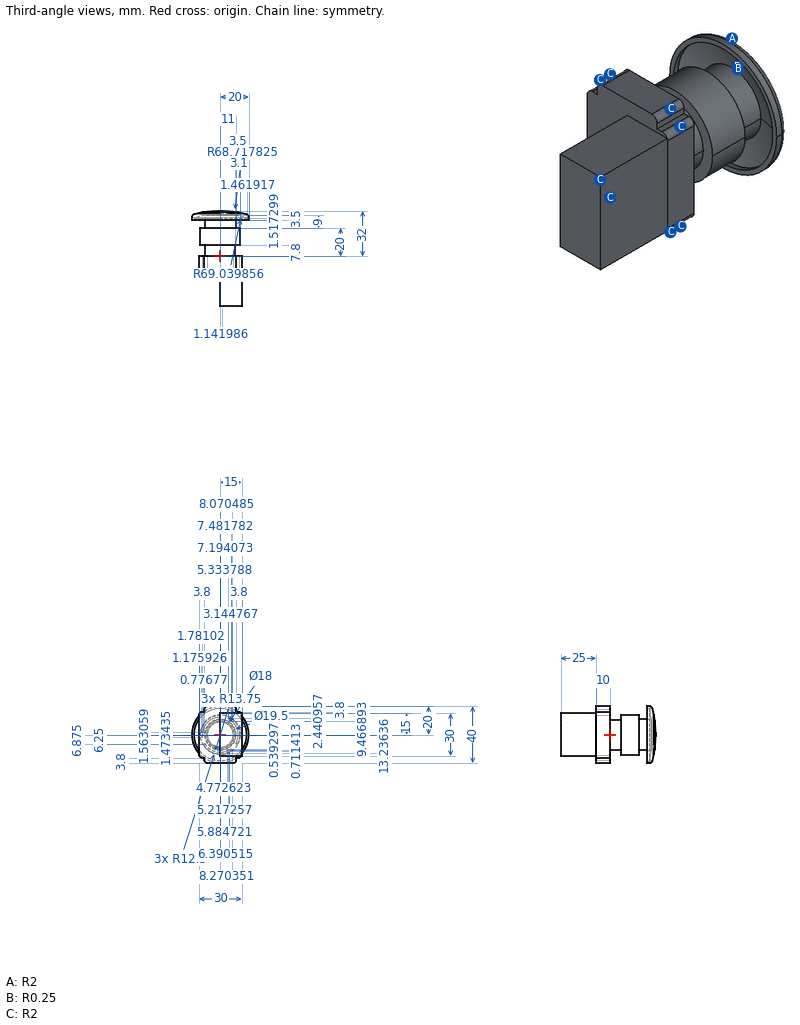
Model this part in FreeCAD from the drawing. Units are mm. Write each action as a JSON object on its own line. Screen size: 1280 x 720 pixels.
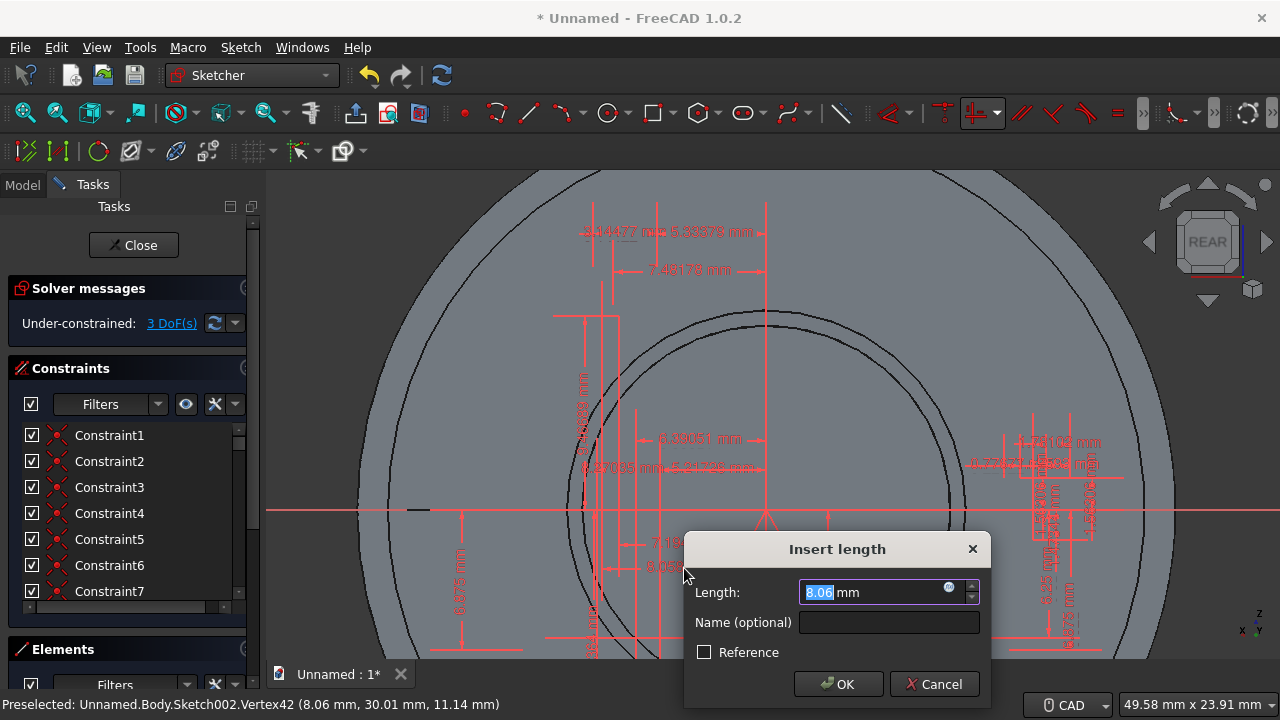
{"action": "type", "text": "8.070485"}
{"action": "key", "text": "Return"}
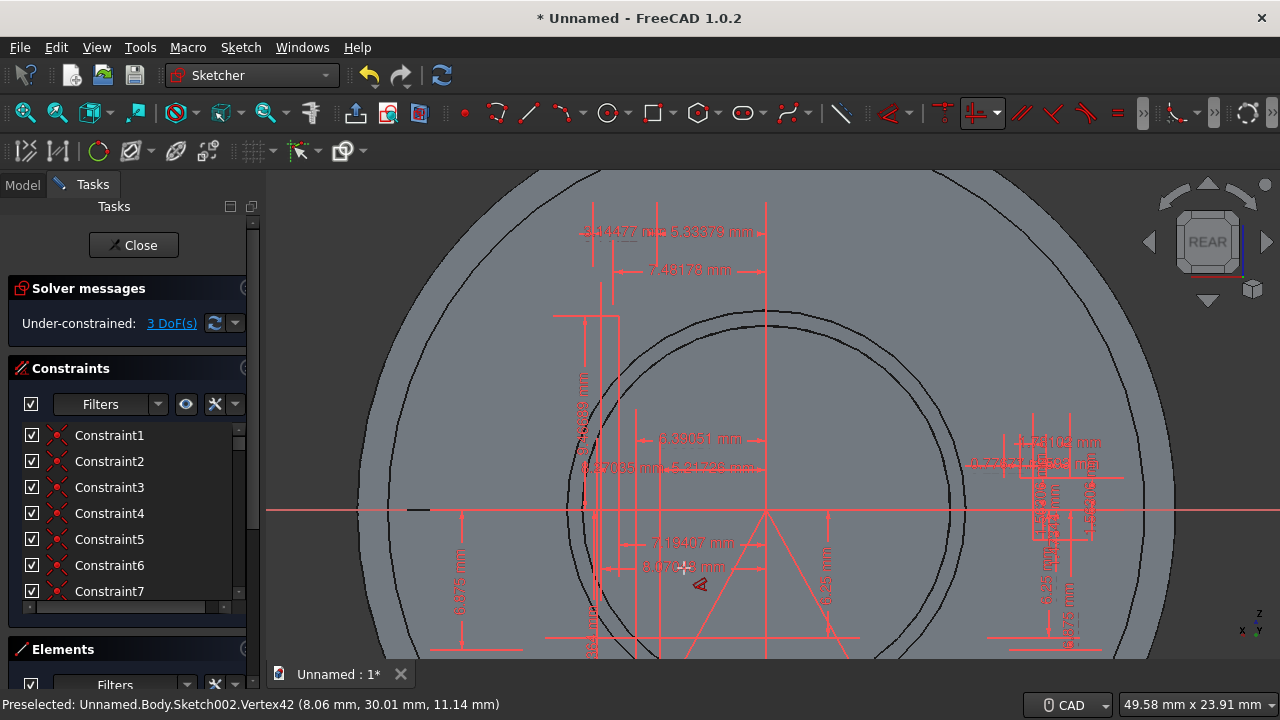
{"action": "scroll", "coordinate": [612, 305], "scroll_direction": "down", "scroll_amount": 3}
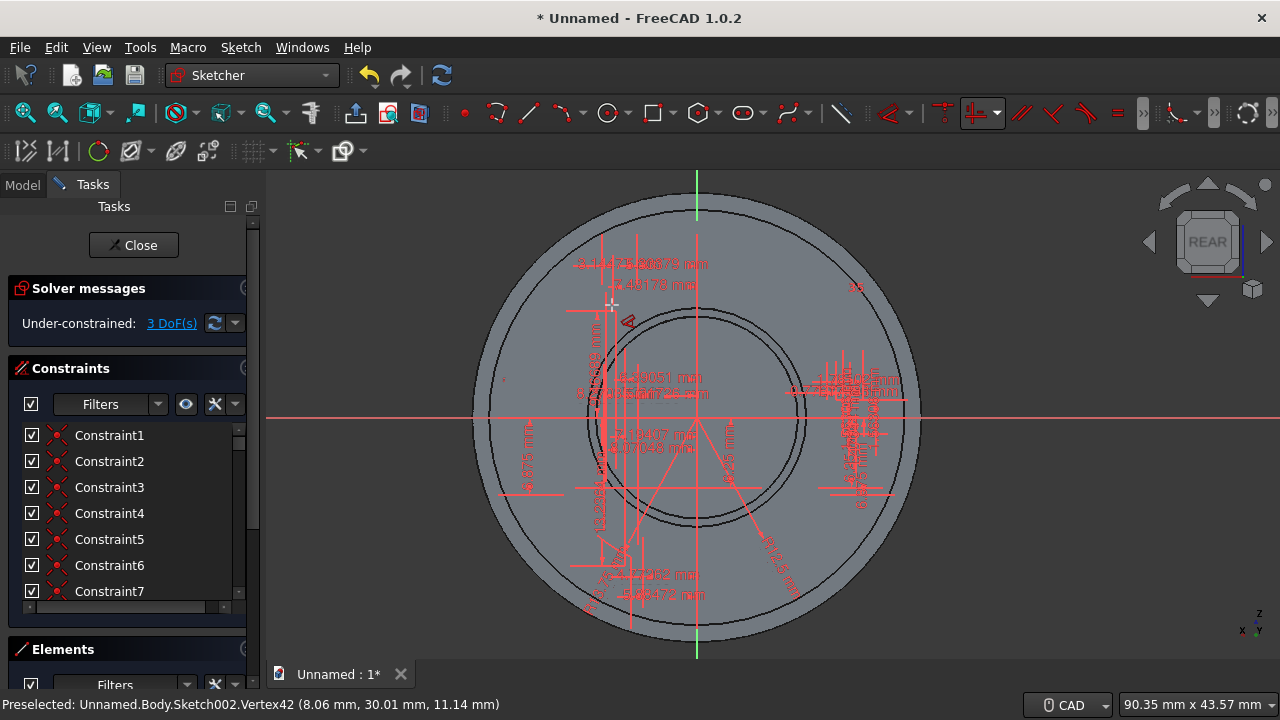
{"action": "scroll", "coordinate": [641, 541], "scroll_direction": "up", "scroll_amount": 9}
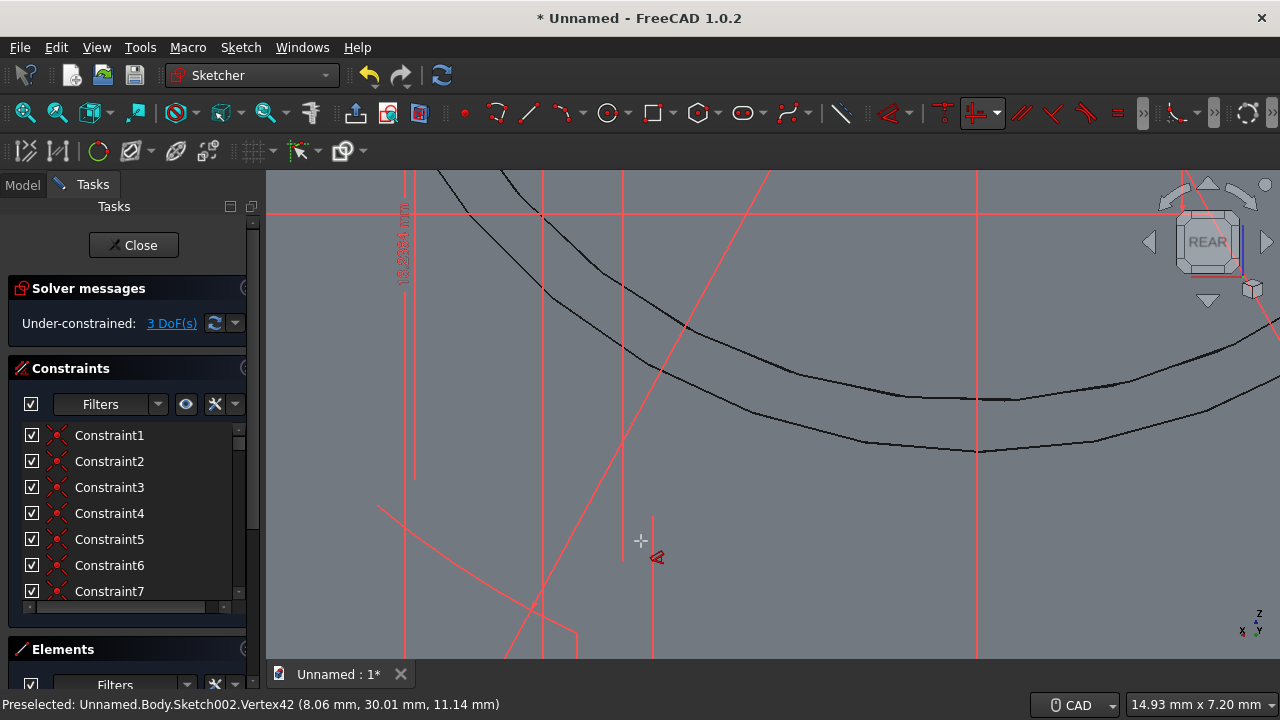
{"action": "left_click", "coordinate": [638, 538]}
{"action": "left_click", "coordinate": [589, 538]}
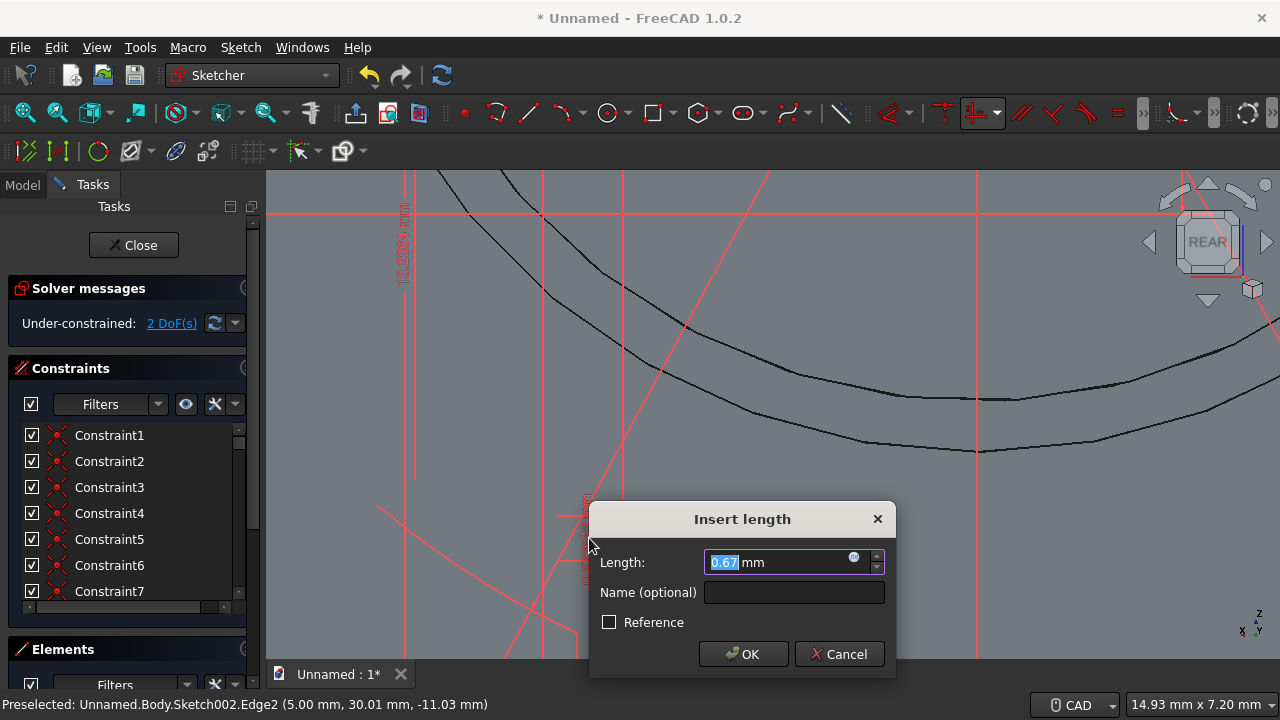
{"action": "type", "text": "0.711413"}
{"action": "key", "text": "Return"}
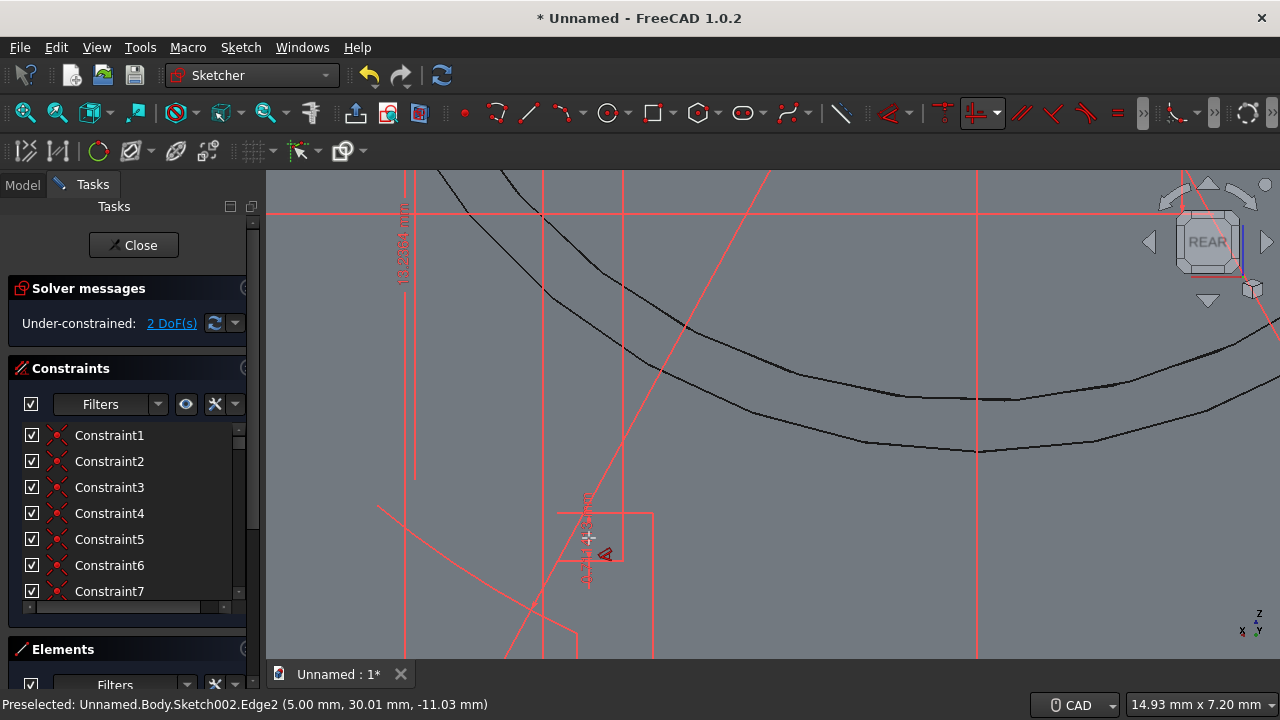
{"action": "left_click", "coordinate": [582, 503]}
{"action": "left_click", "coordinate": [381, 496]}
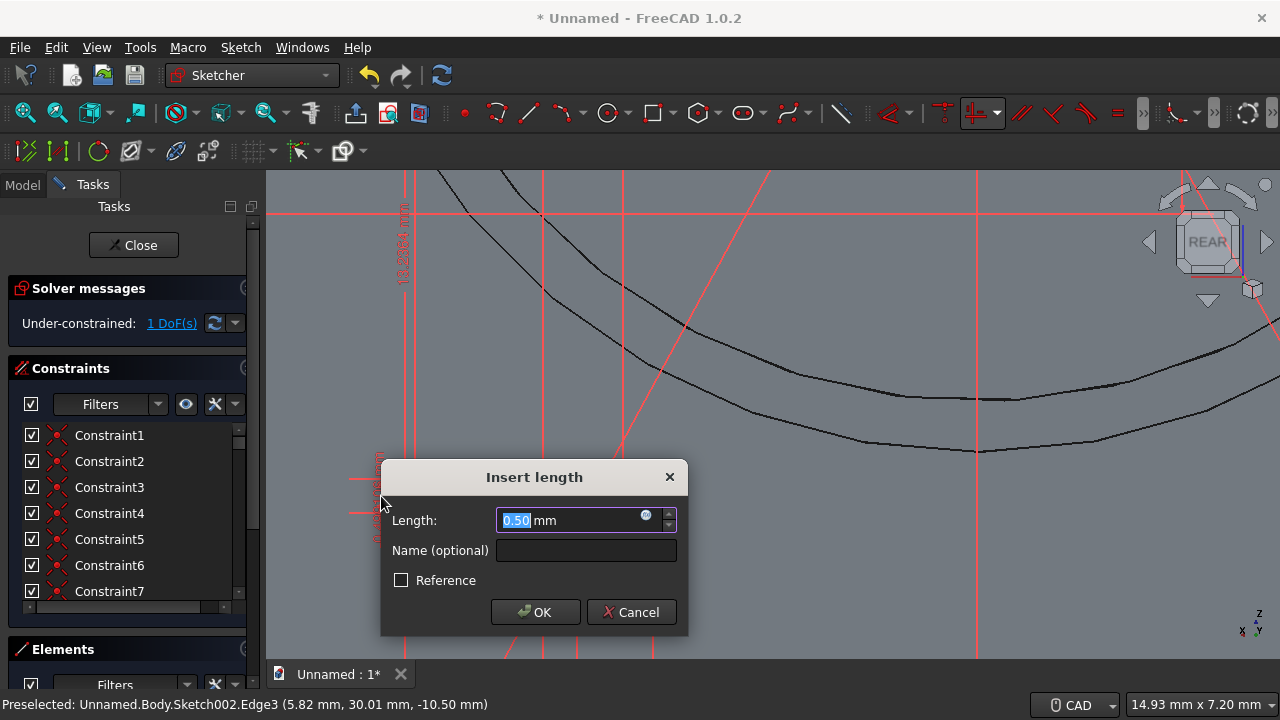
{"action": "type", "text": "0.539297"}
{"action": "key", "text": "Return"}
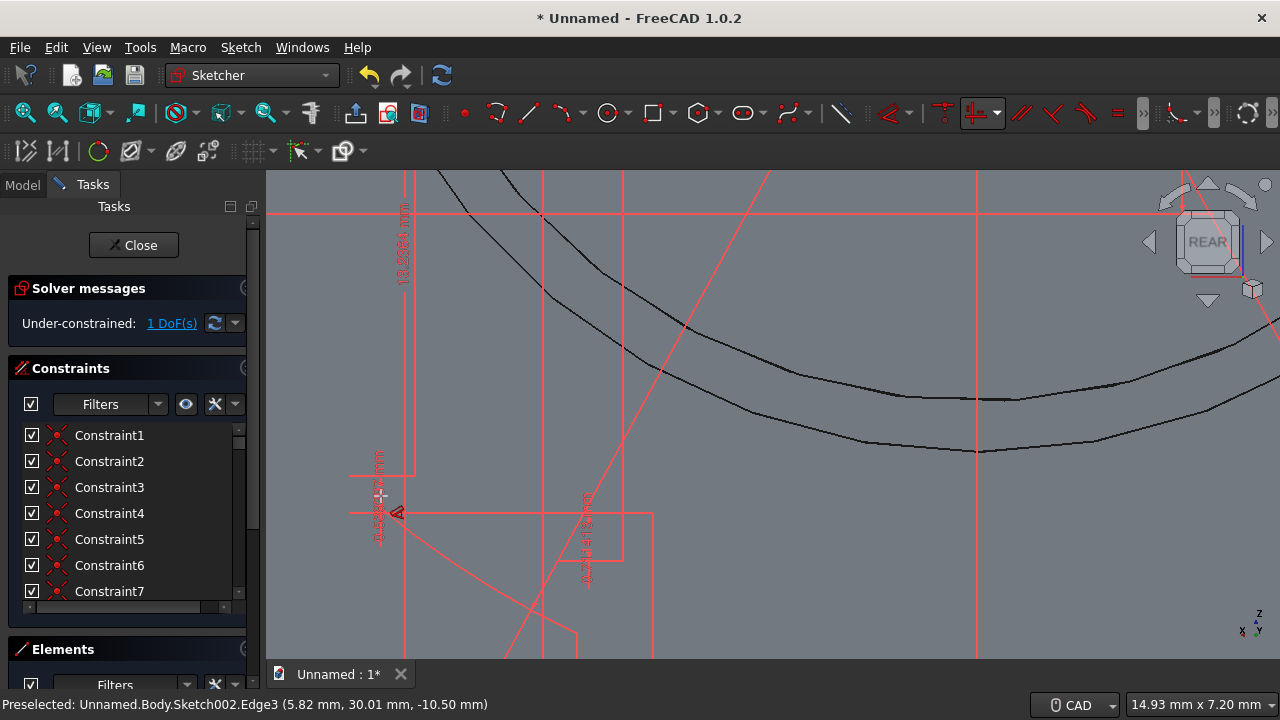
{"action": "scroll", "coordinate": [641, 542], "scroll_direction": "down", "scroll_amount": 9}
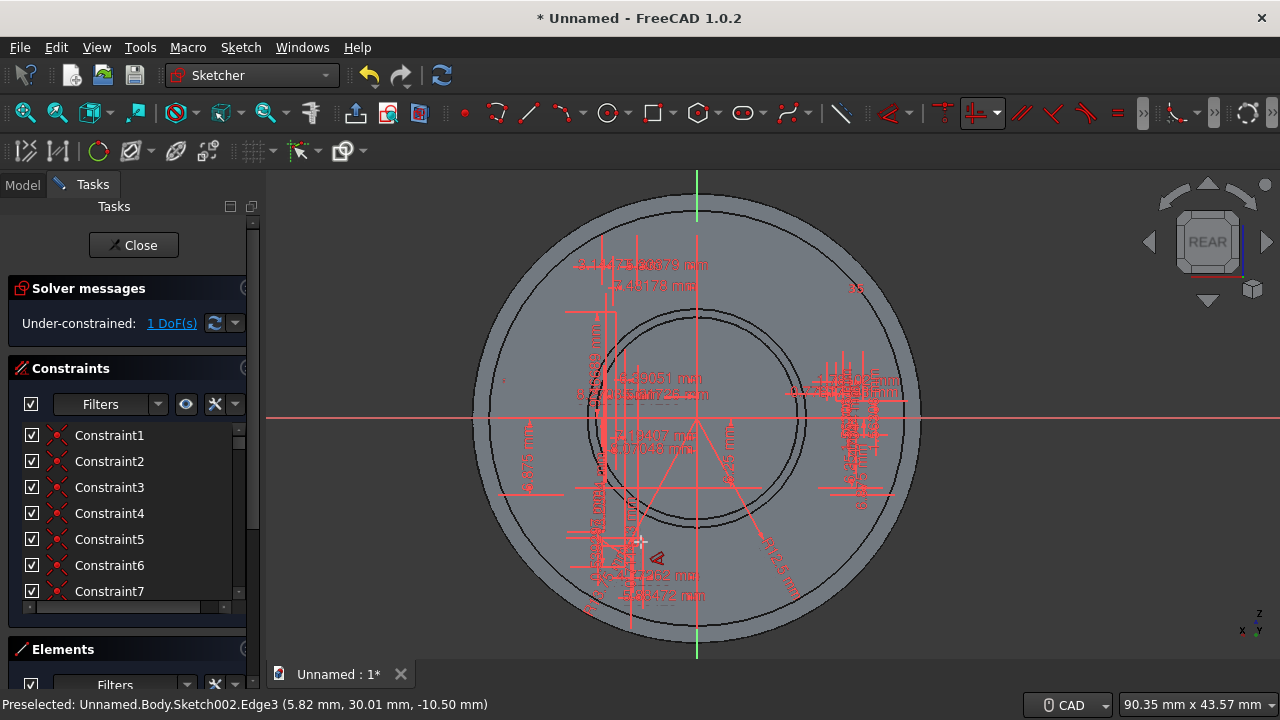
{"action": "scroll", "coordinate": [622, 304], "scroll_direction": "up", "scroll_amount": 2}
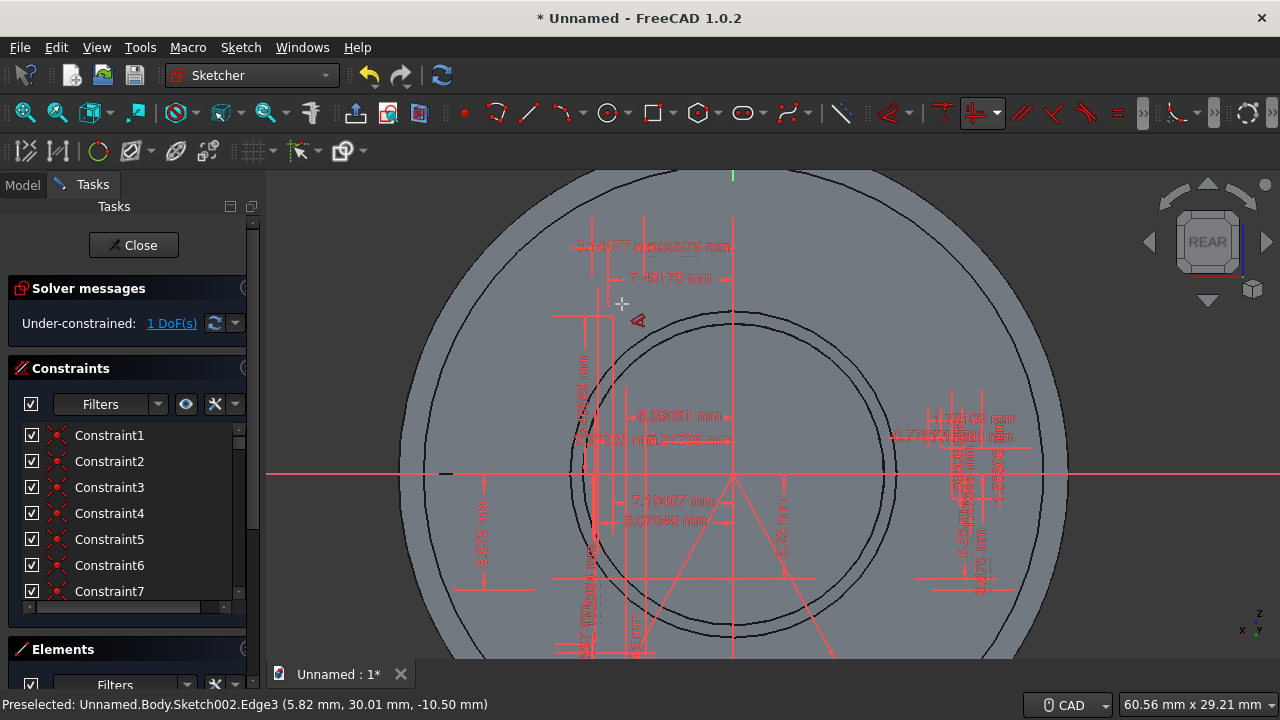
{"action": "left_click", "coordinate": [622, 304]}
{"action": "left_click", "coordinate": [579, 286]}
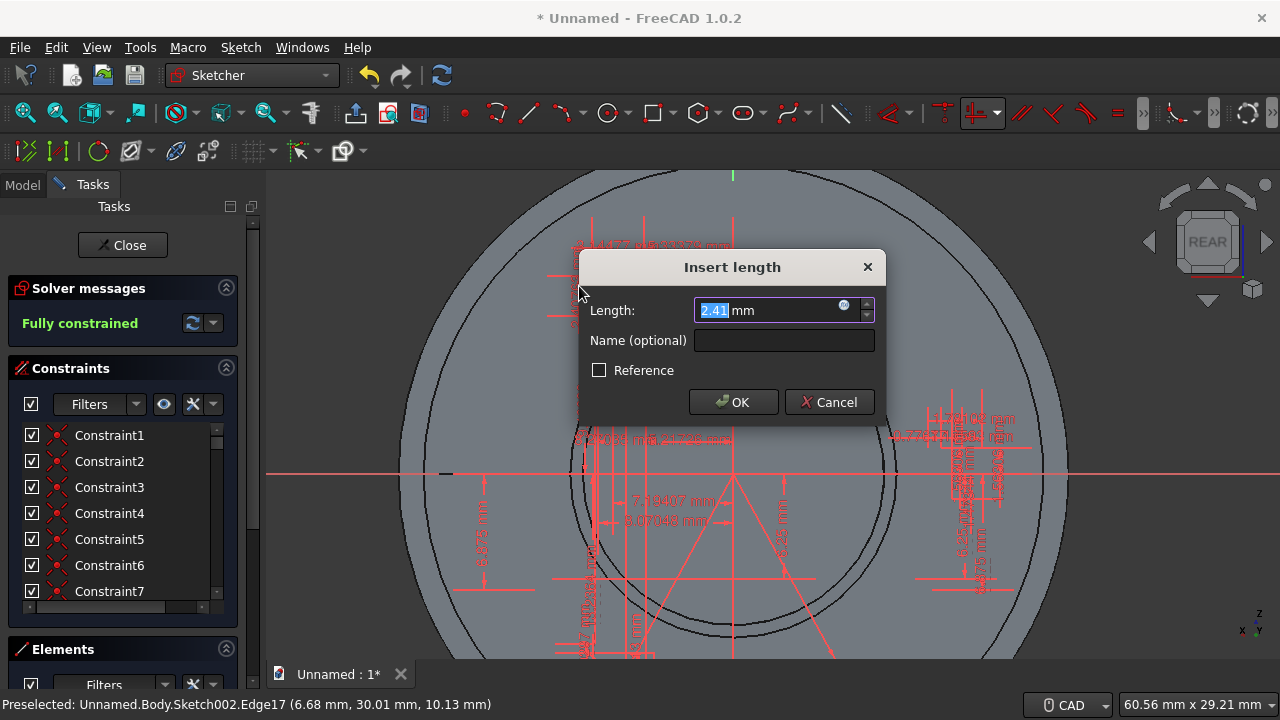
{"action": "type", "text": "2.440957"}
{"action": "key", "text": "Return"}
{"action": "key", "text": "Escape"}